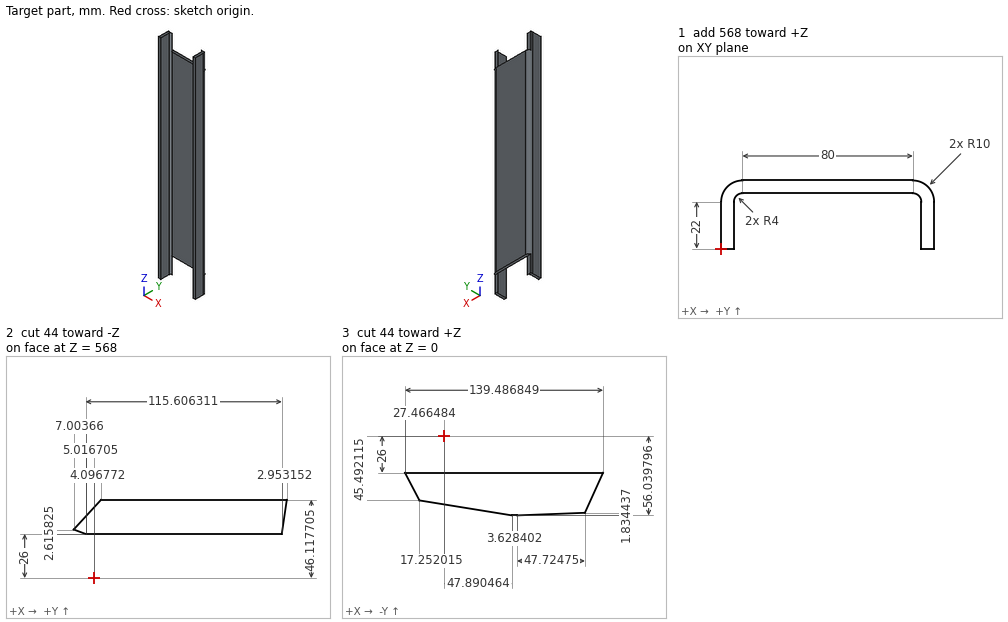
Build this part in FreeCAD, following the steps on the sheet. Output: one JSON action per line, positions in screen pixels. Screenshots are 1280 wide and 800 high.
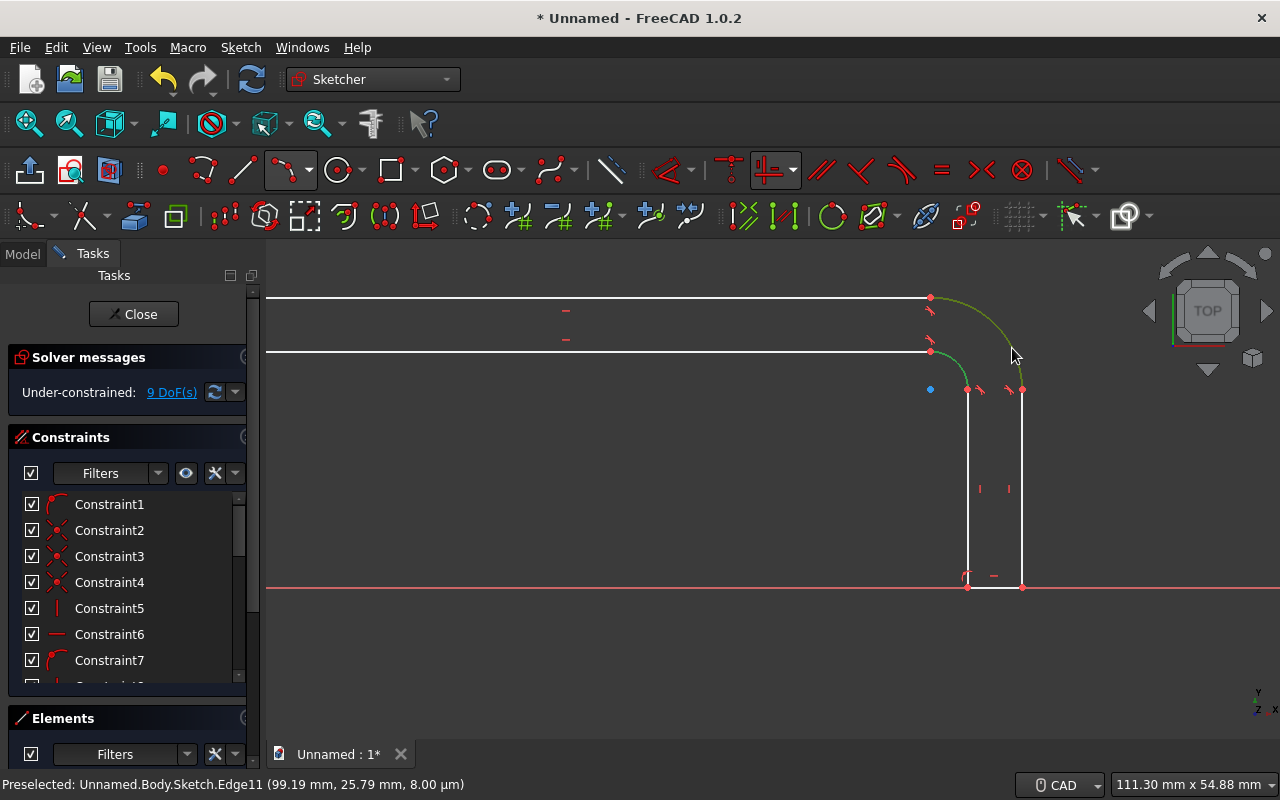
{"action": "left_click", "coordinate": [730, 170]}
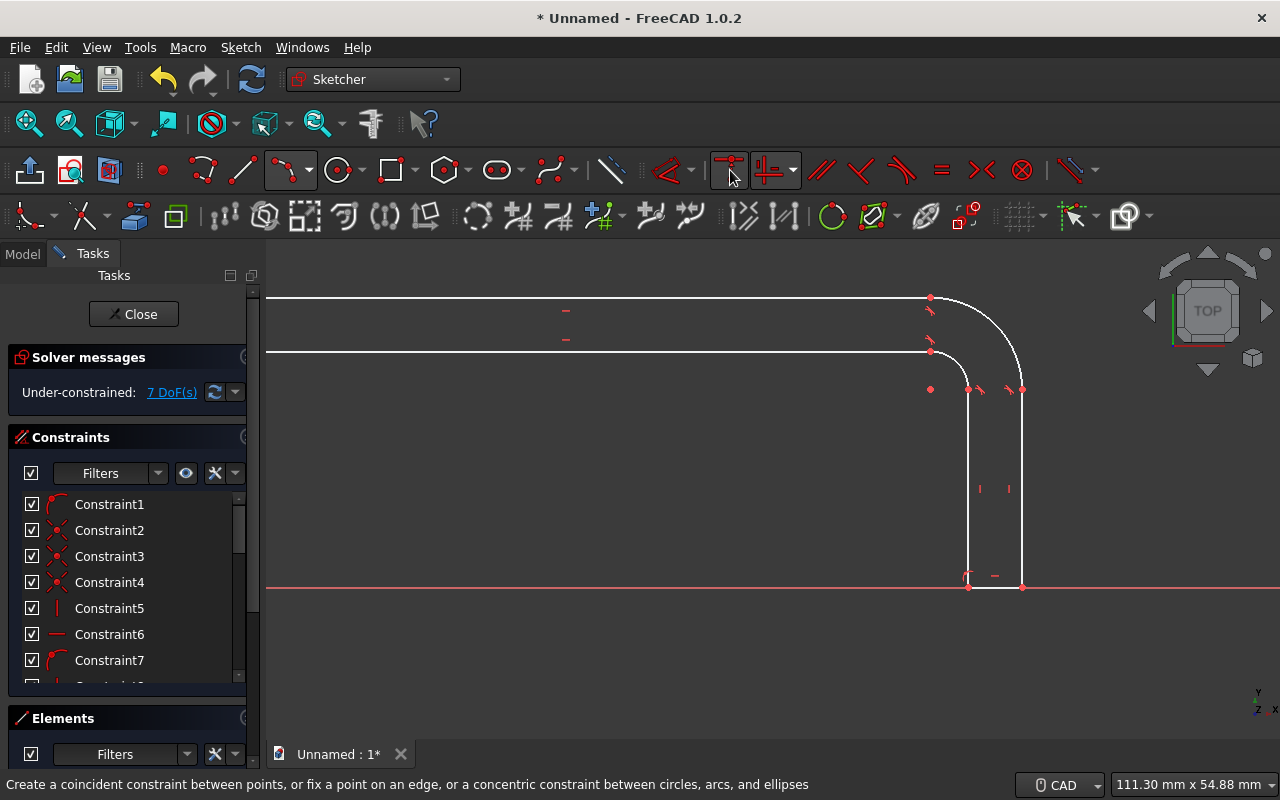
{"action": "scroll", "coordinate": [985, 585], "scroll_direction": "down", "scroll_amount": 2}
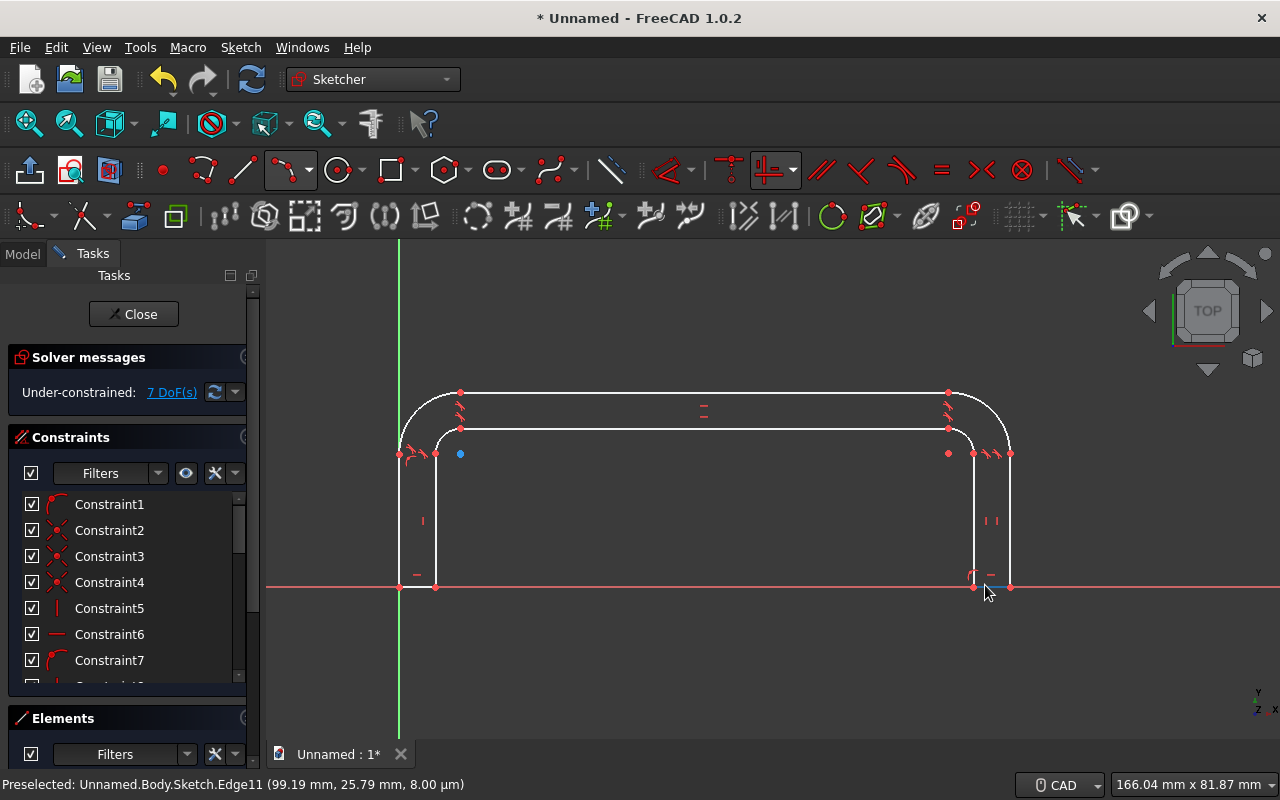
{"action": "left_click", "coordinate": [449, 431]}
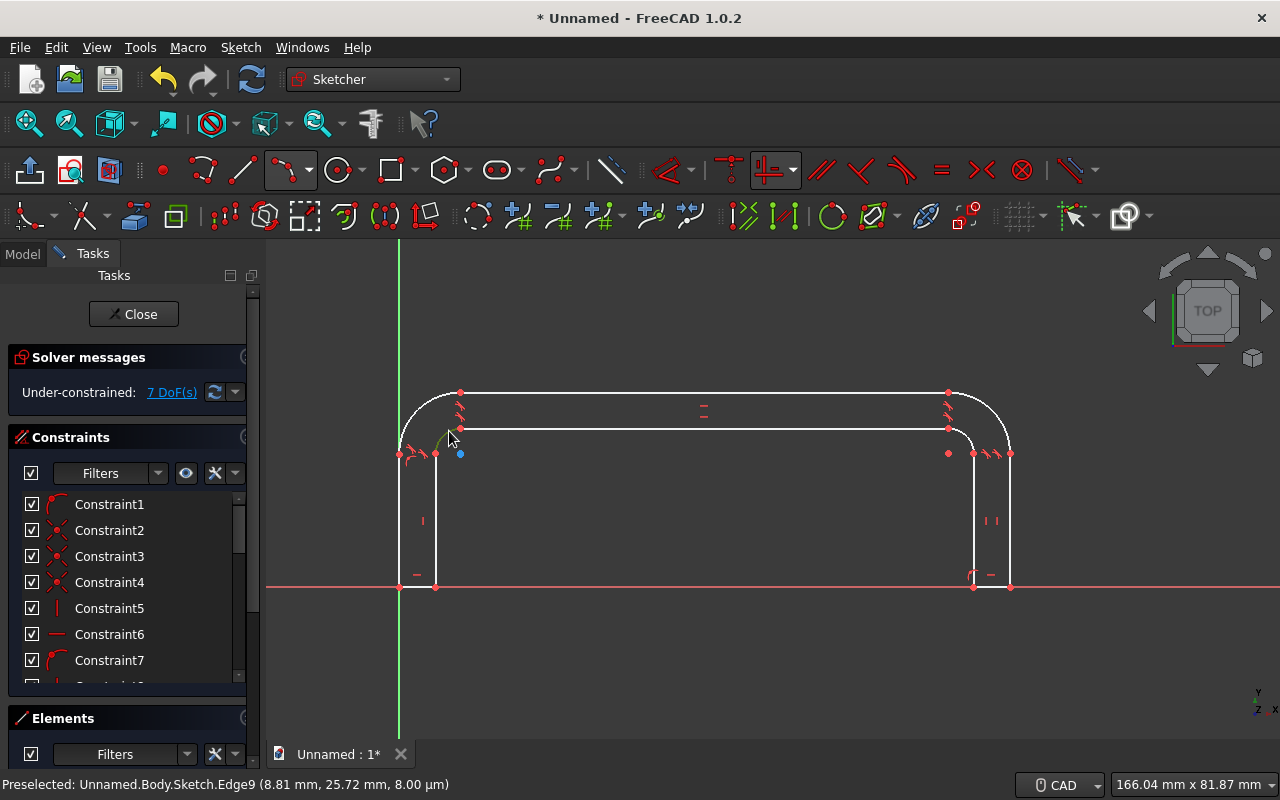
{"action": "left_click", "coordinate": [433, 399]}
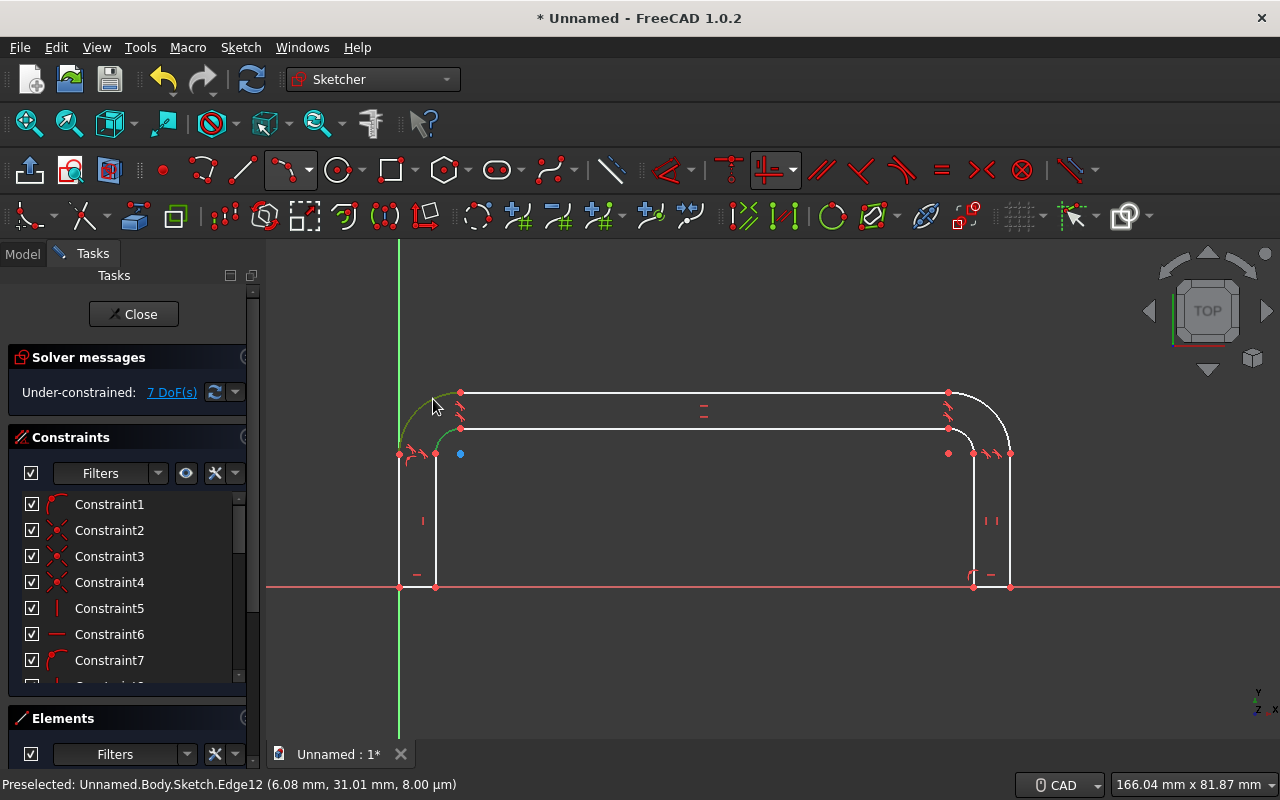
{"action": "left_click", "coordinate": [730, 170]}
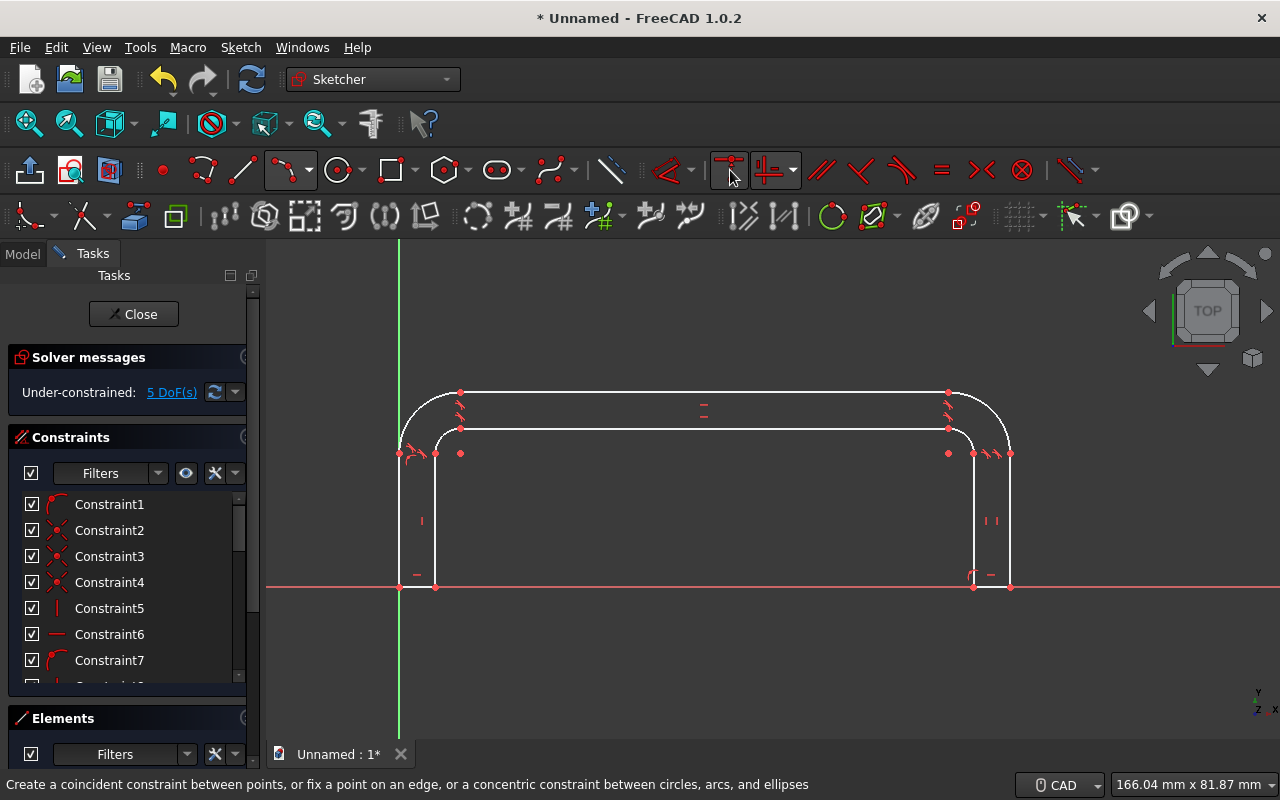
{"action": "left_click", "coordinate": [449, 431]}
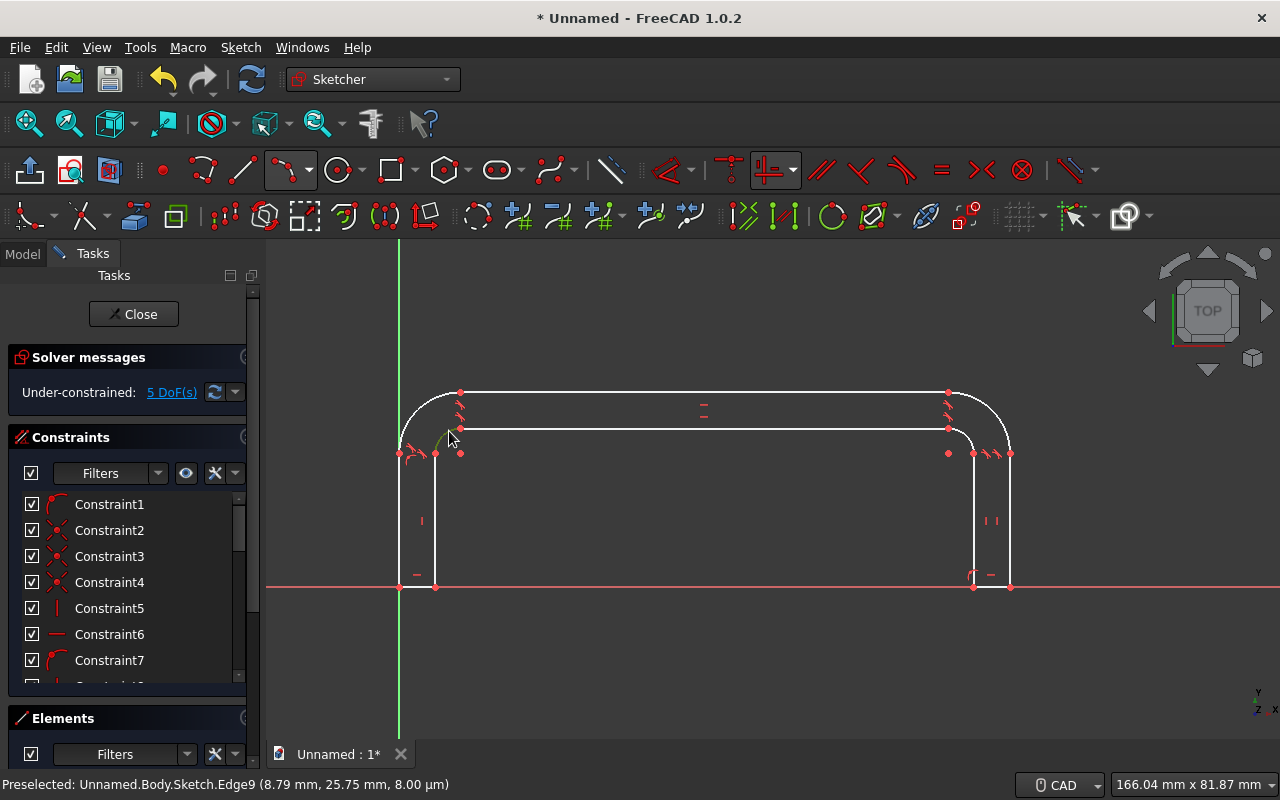
{"action": "left_click", "coordinate": [971, 442]}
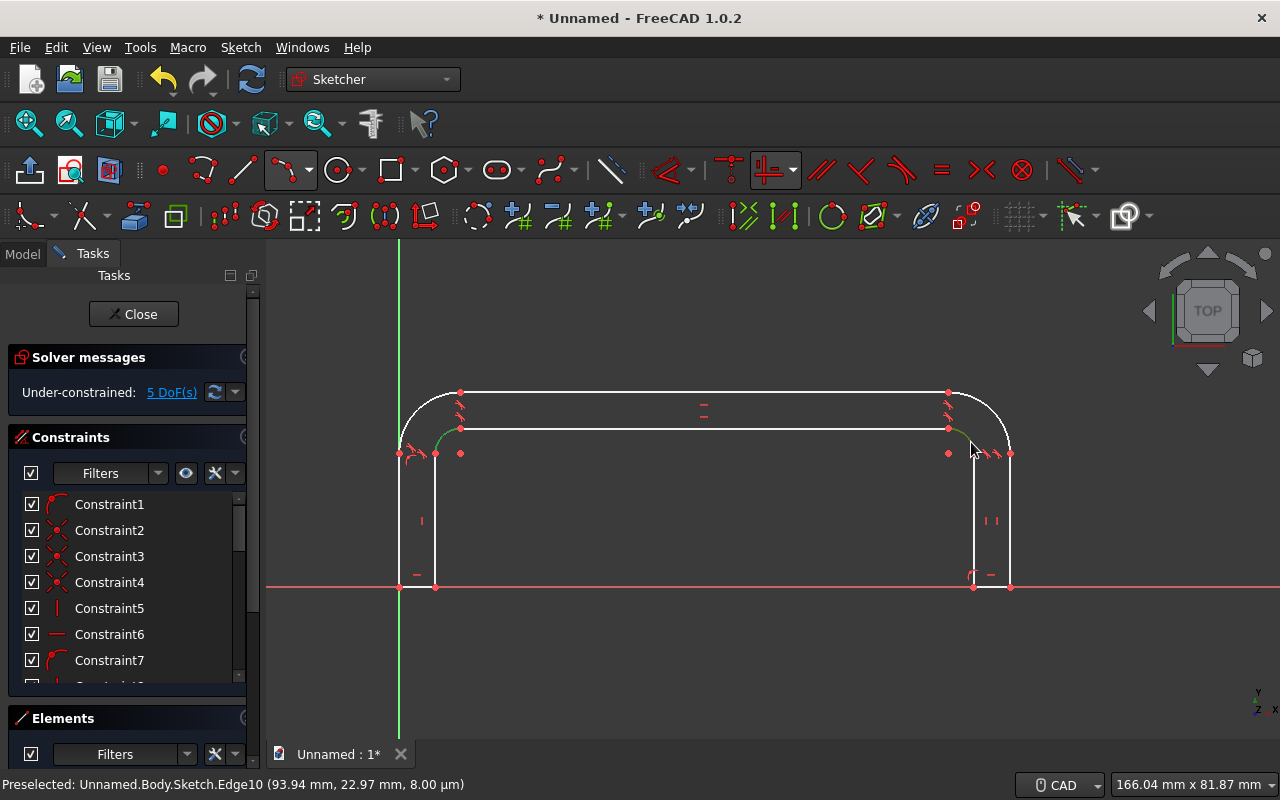
{"action": "left_click", "coordinate": [942, 170]}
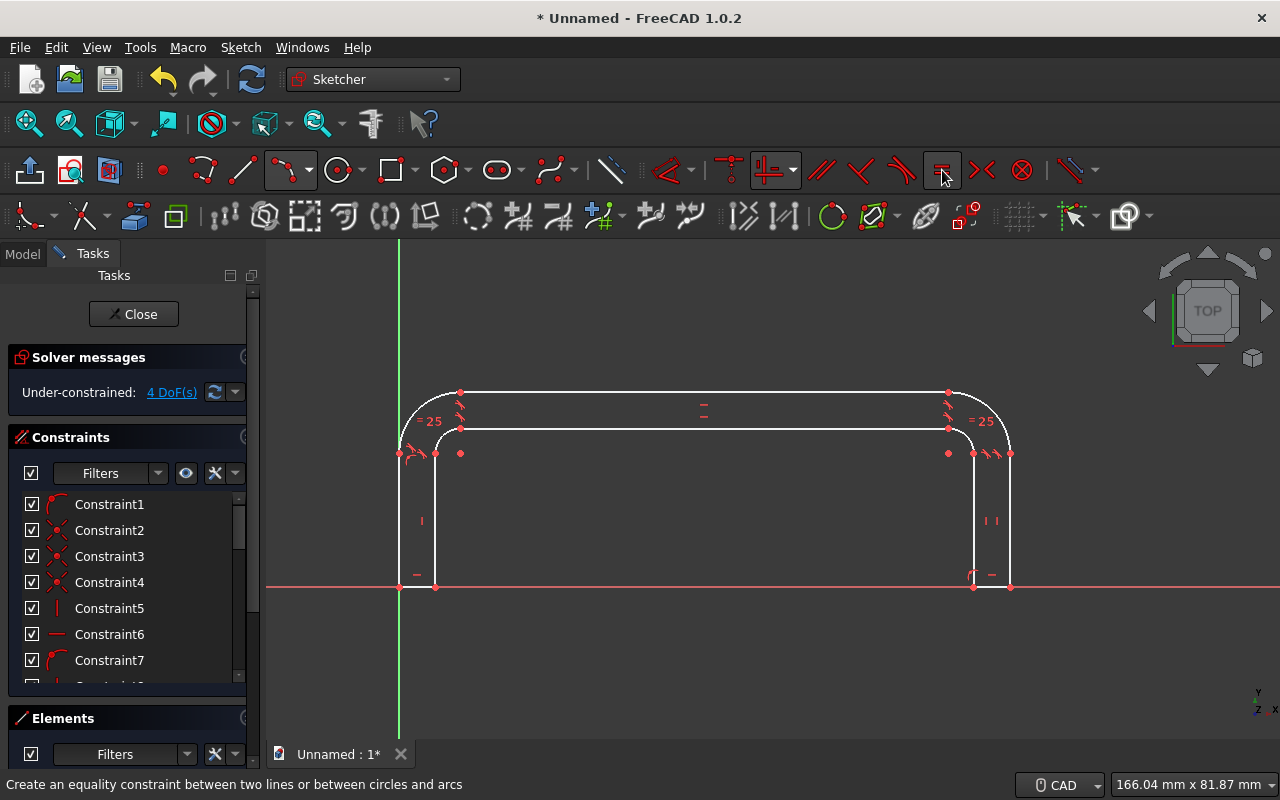
{"action": "scroll", "coordinate": [449, 431], "scroll_direction": "up", "scroll_amount": 3}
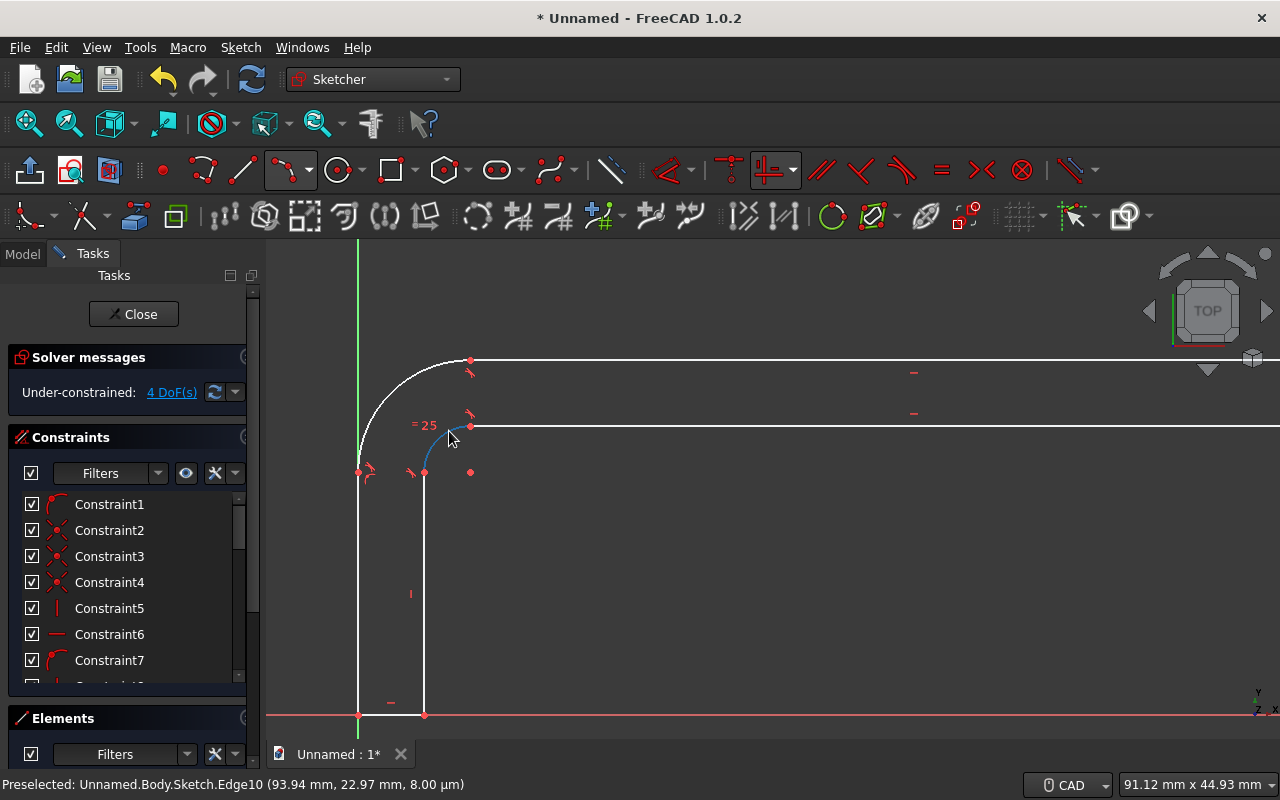
{"action": "left_click", "coordinate": [449, 431]}